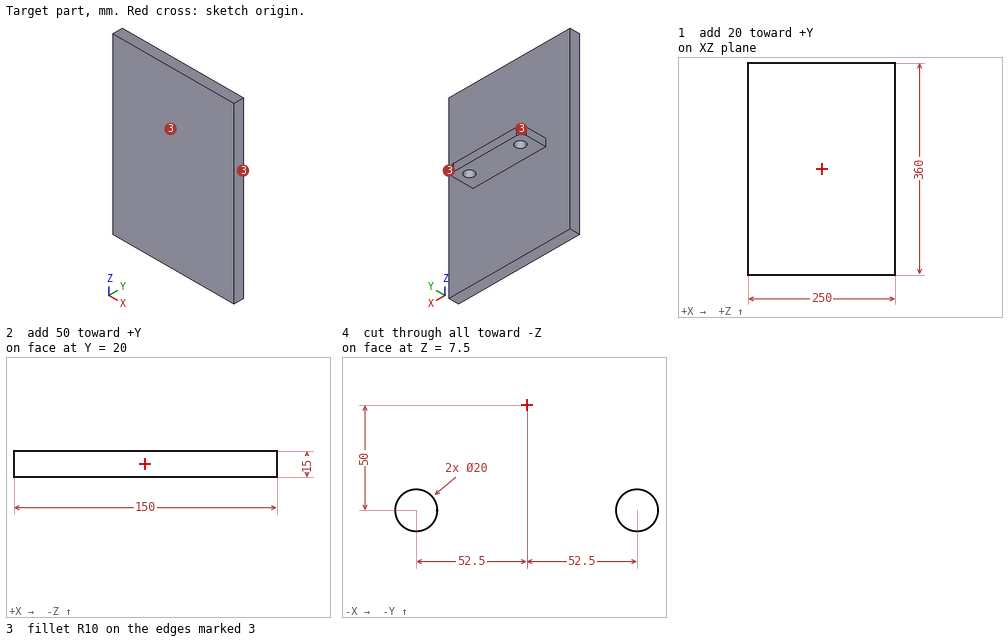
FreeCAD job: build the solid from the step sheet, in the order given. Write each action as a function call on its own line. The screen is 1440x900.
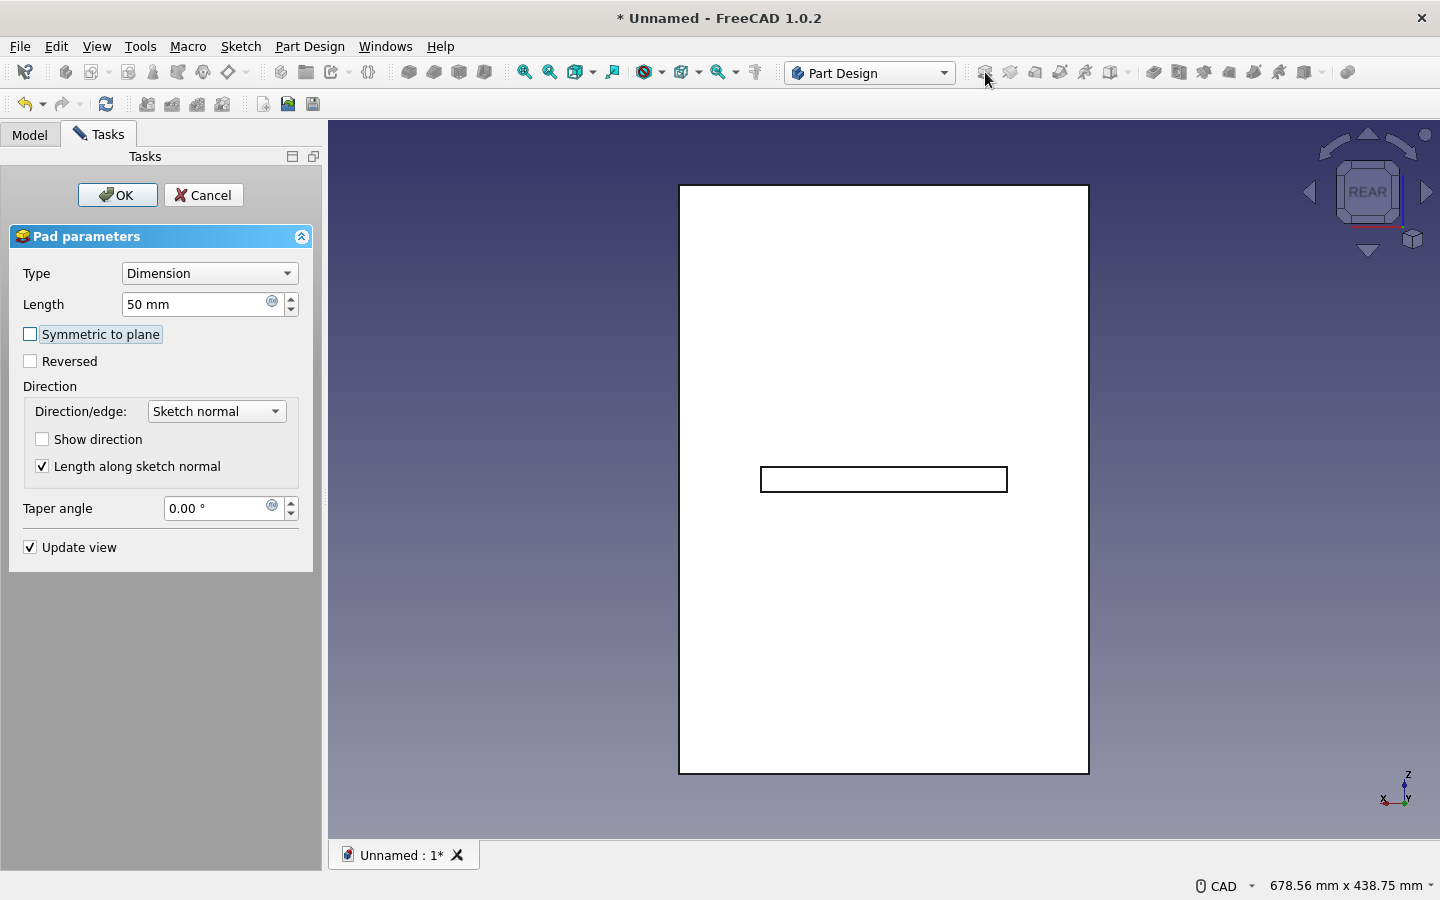
click(118, 195)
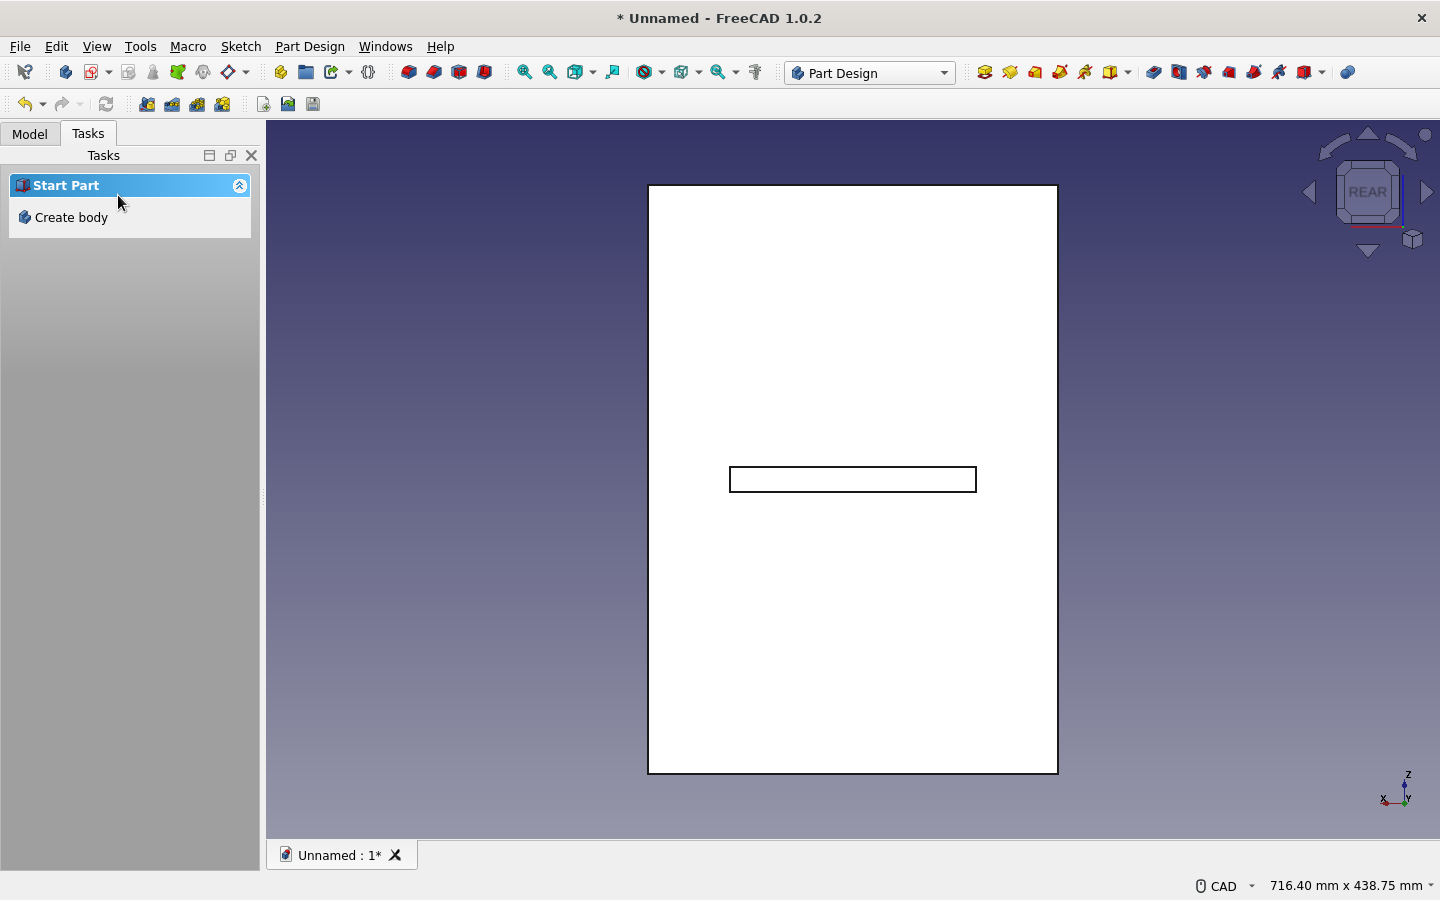
click(976, 479)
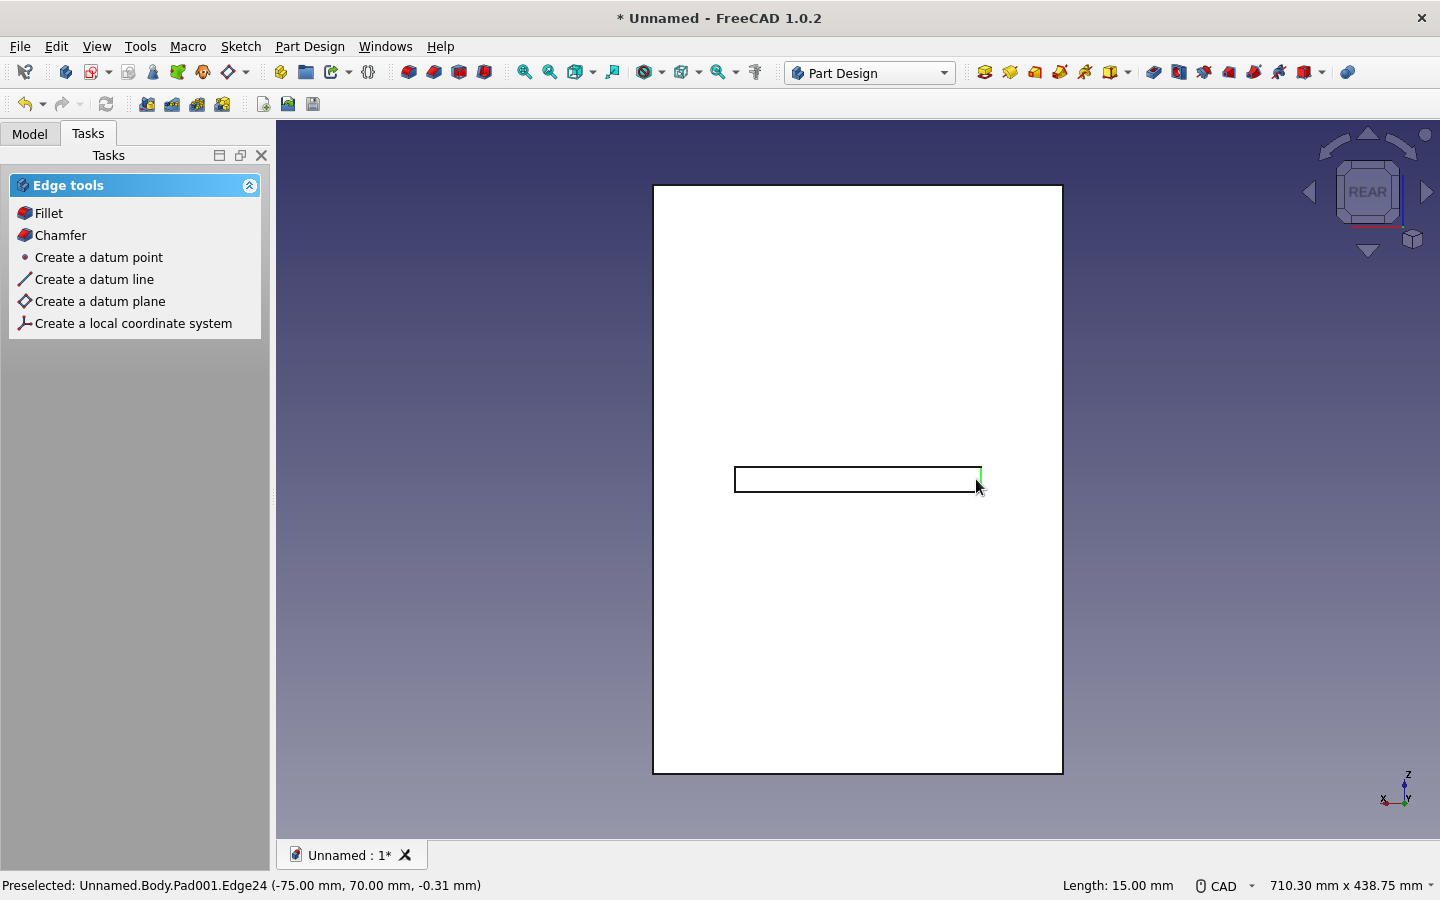
key(0)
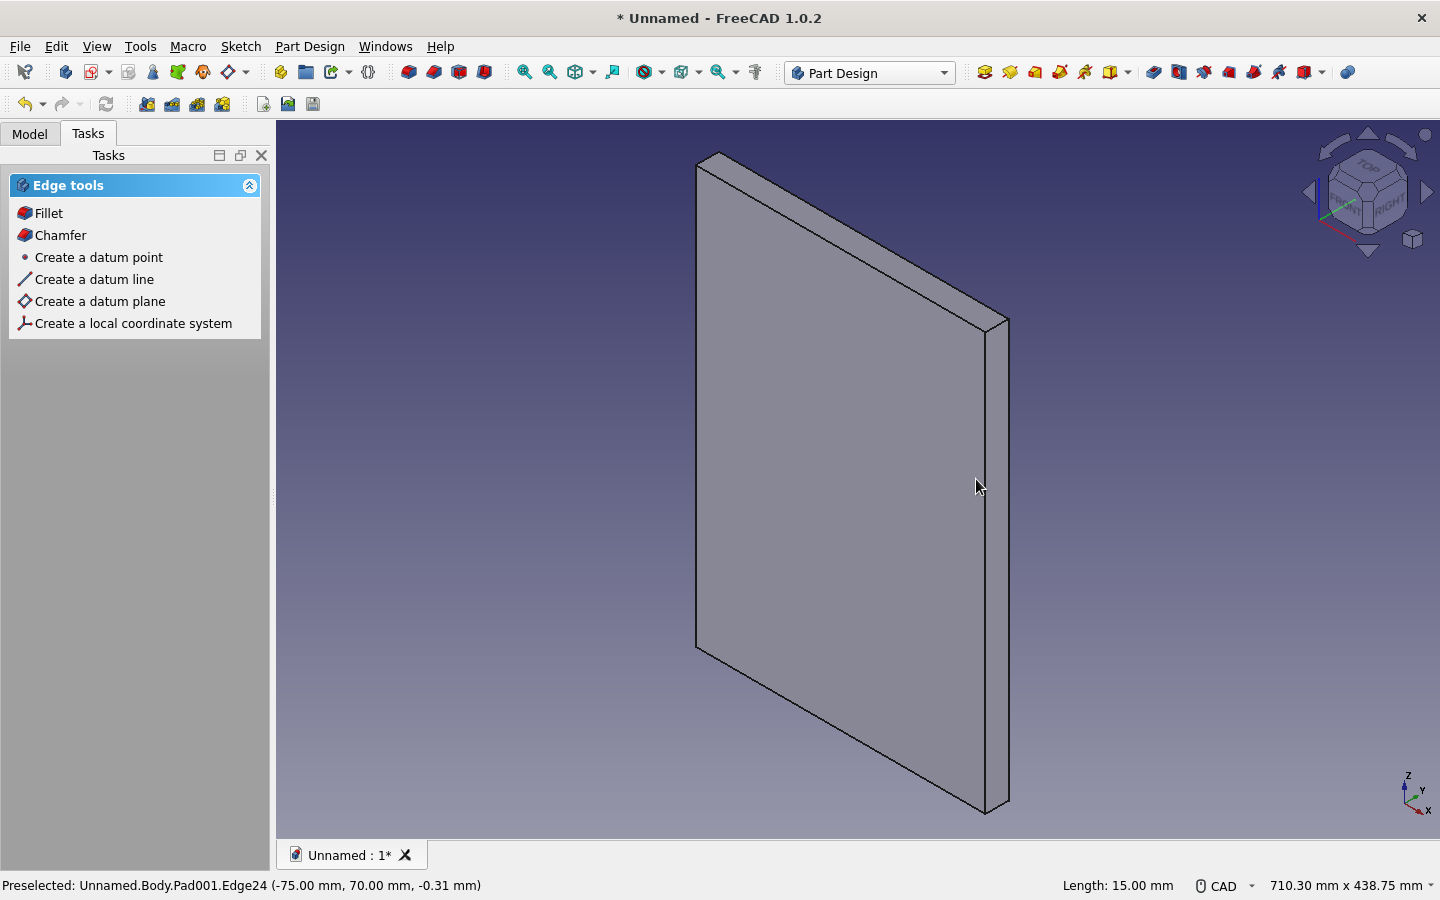
key(v)
key(f)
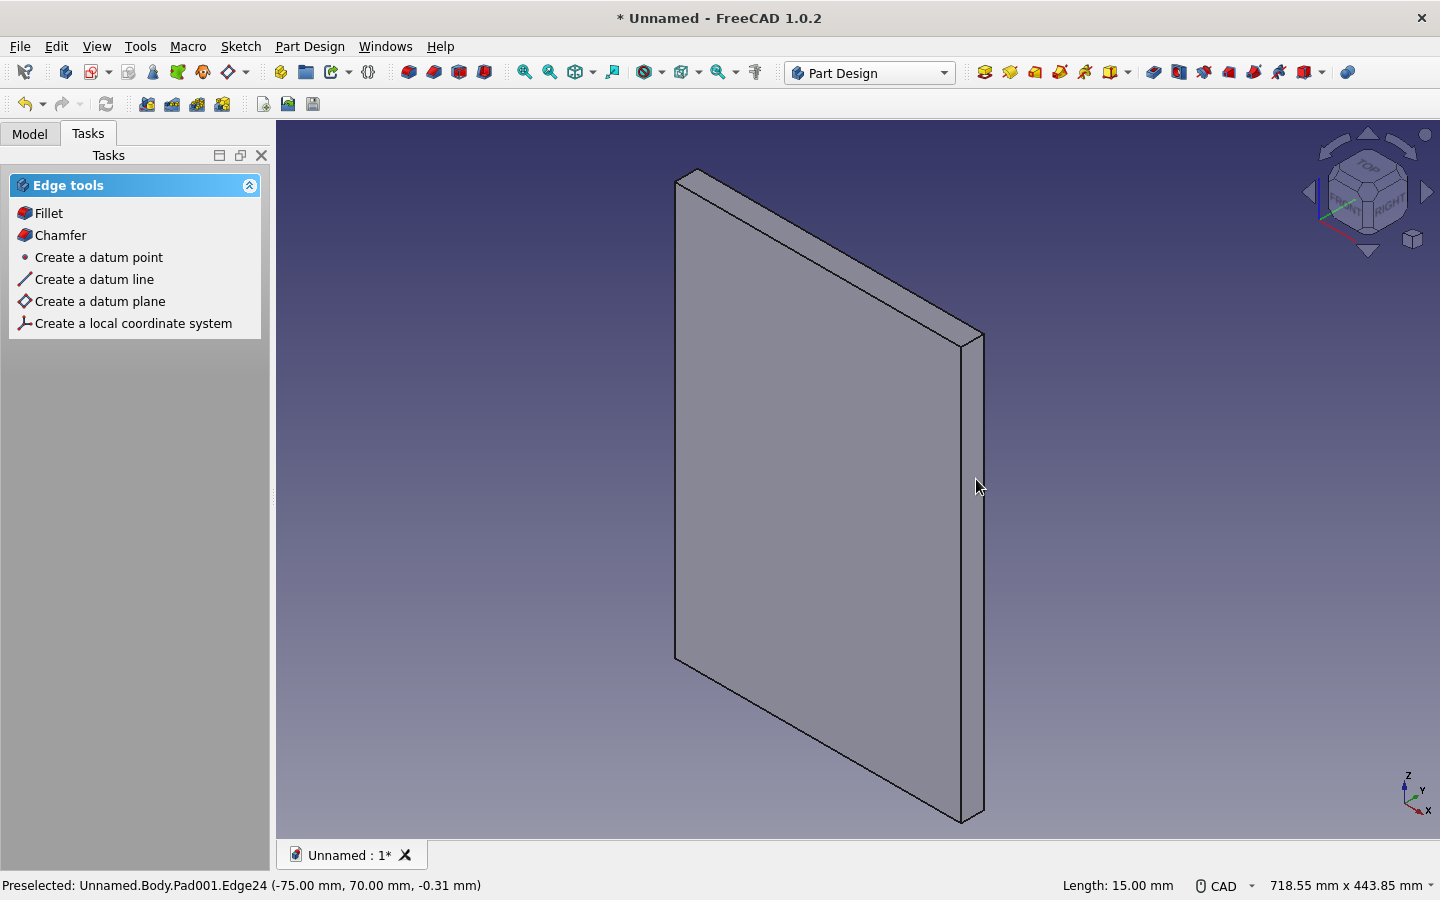
key(2)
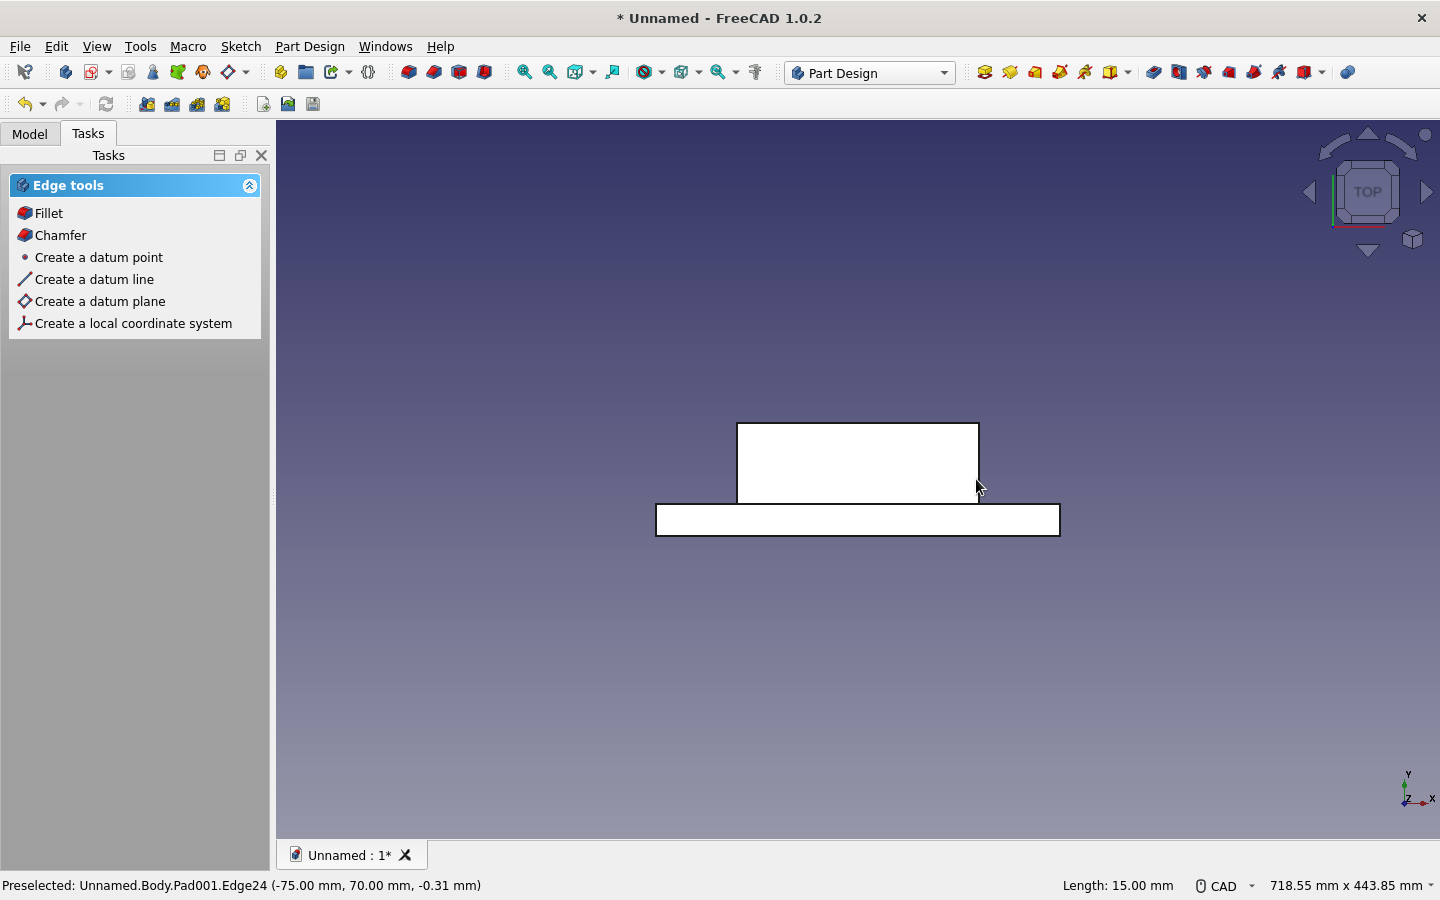
key(v)
key(f)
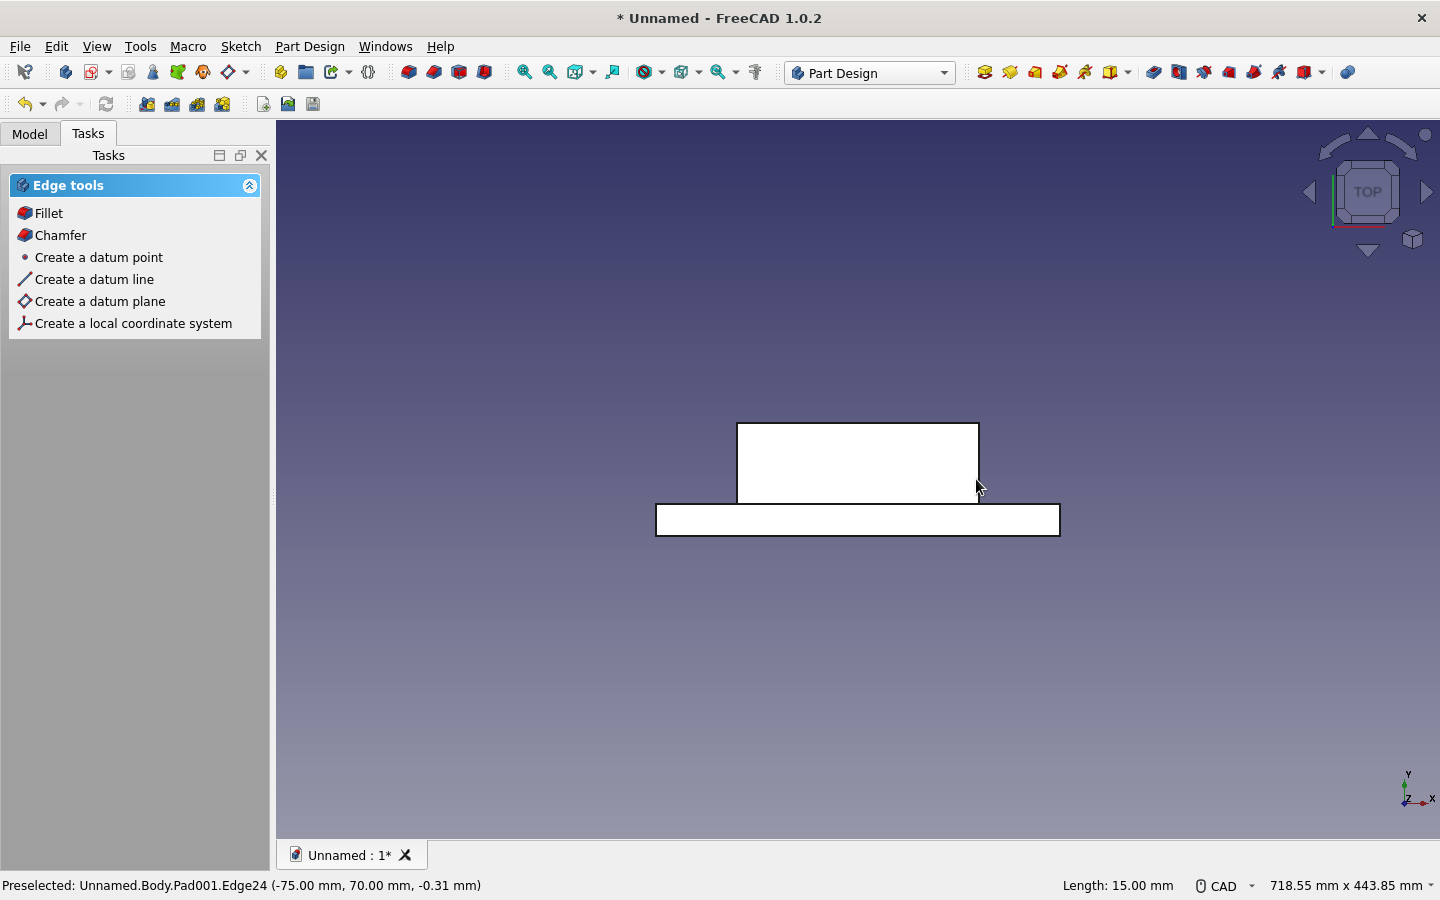
key(1)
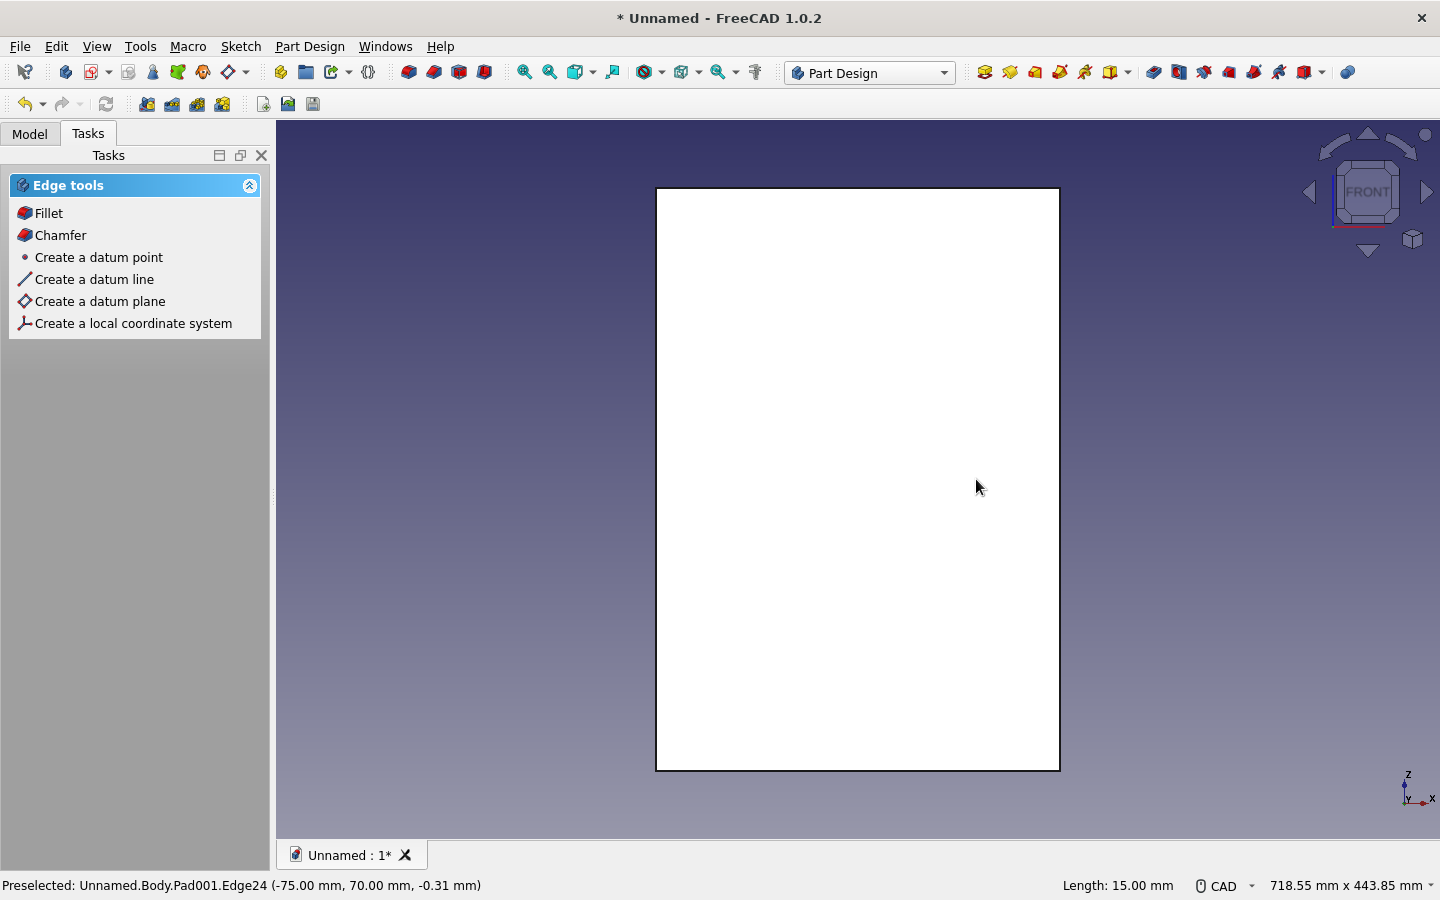
key(3)